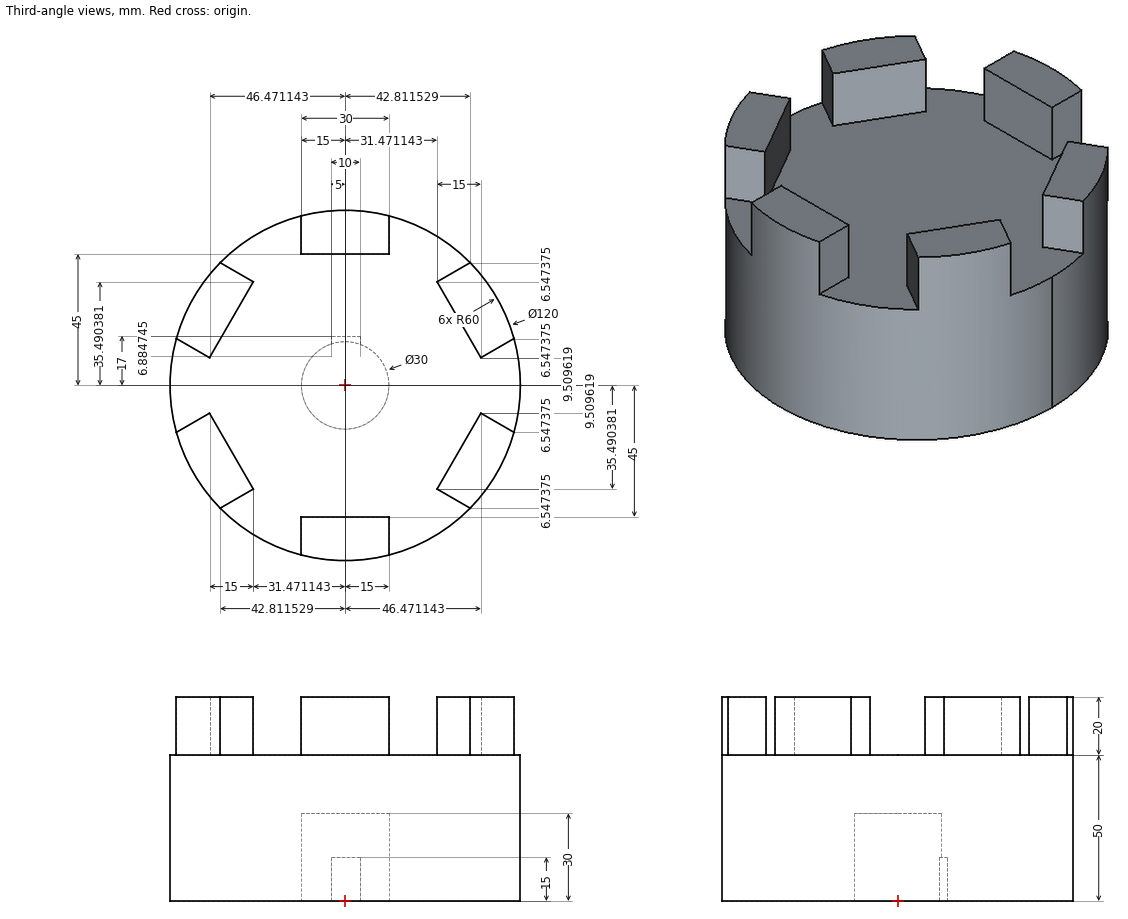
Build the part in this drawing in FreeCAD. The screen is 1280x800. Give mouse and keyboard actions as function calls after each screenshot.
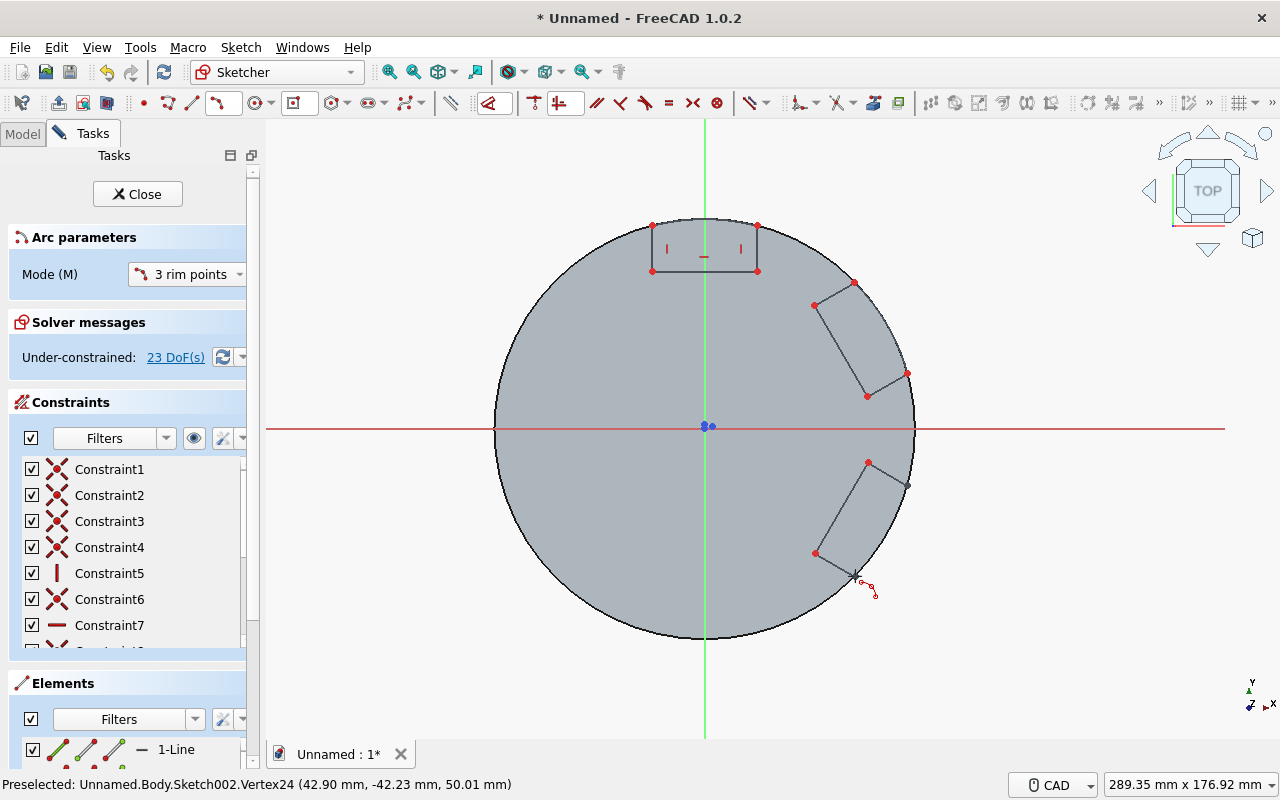
click(855, 577)
click(907, 486)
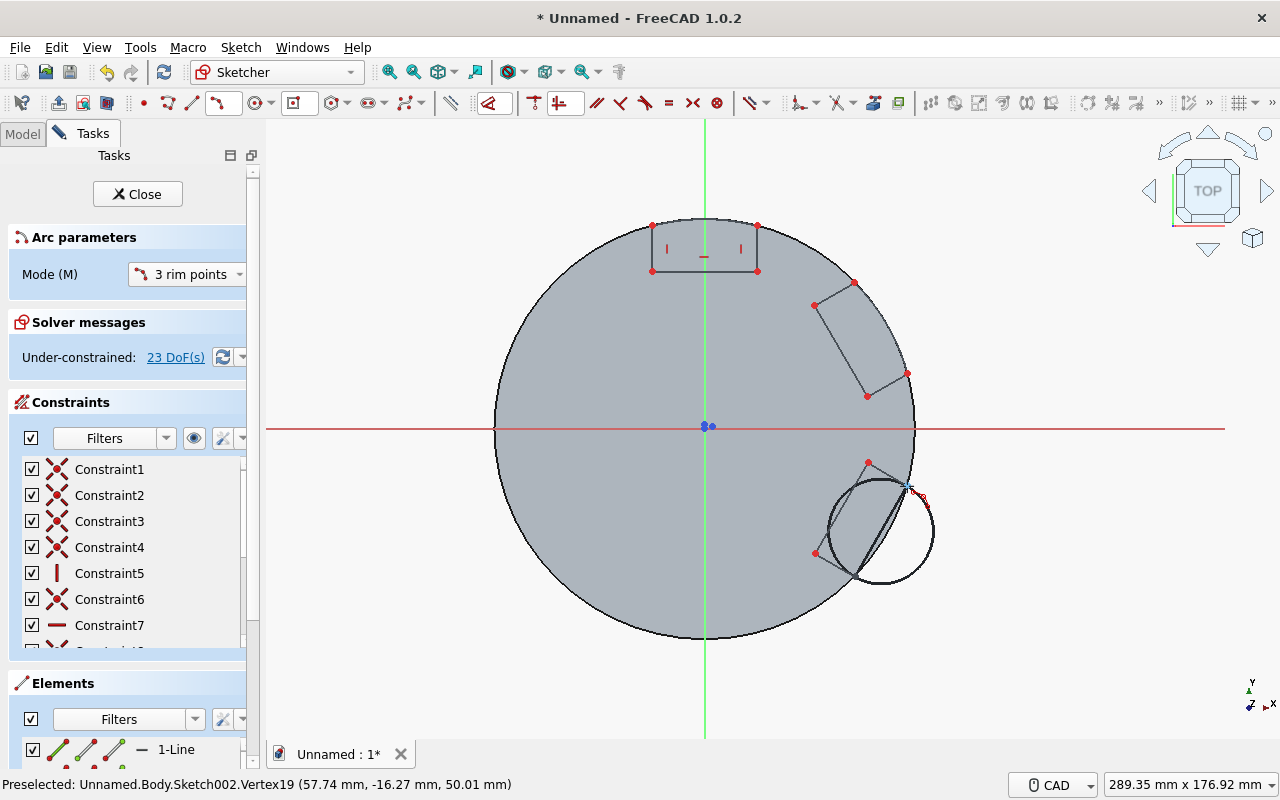
scroll(887, 534, up, 5)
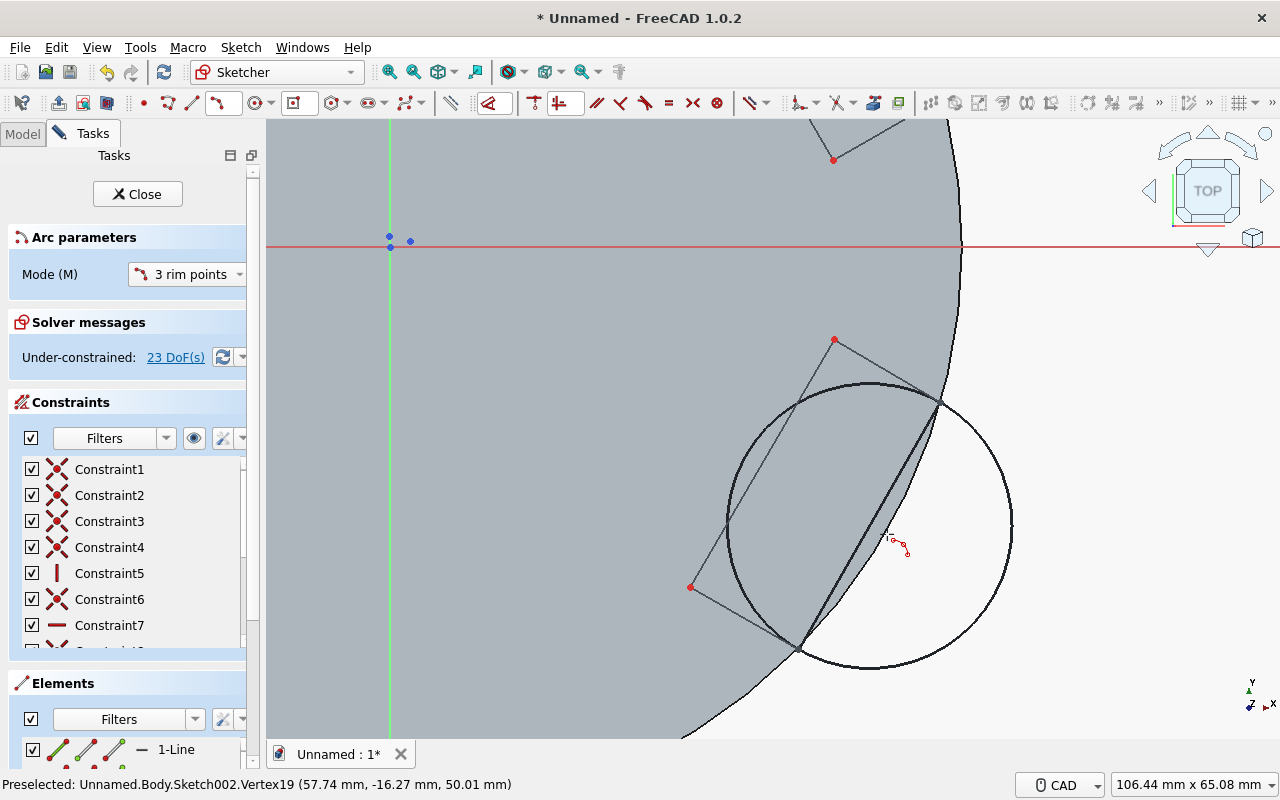
click(885, 533)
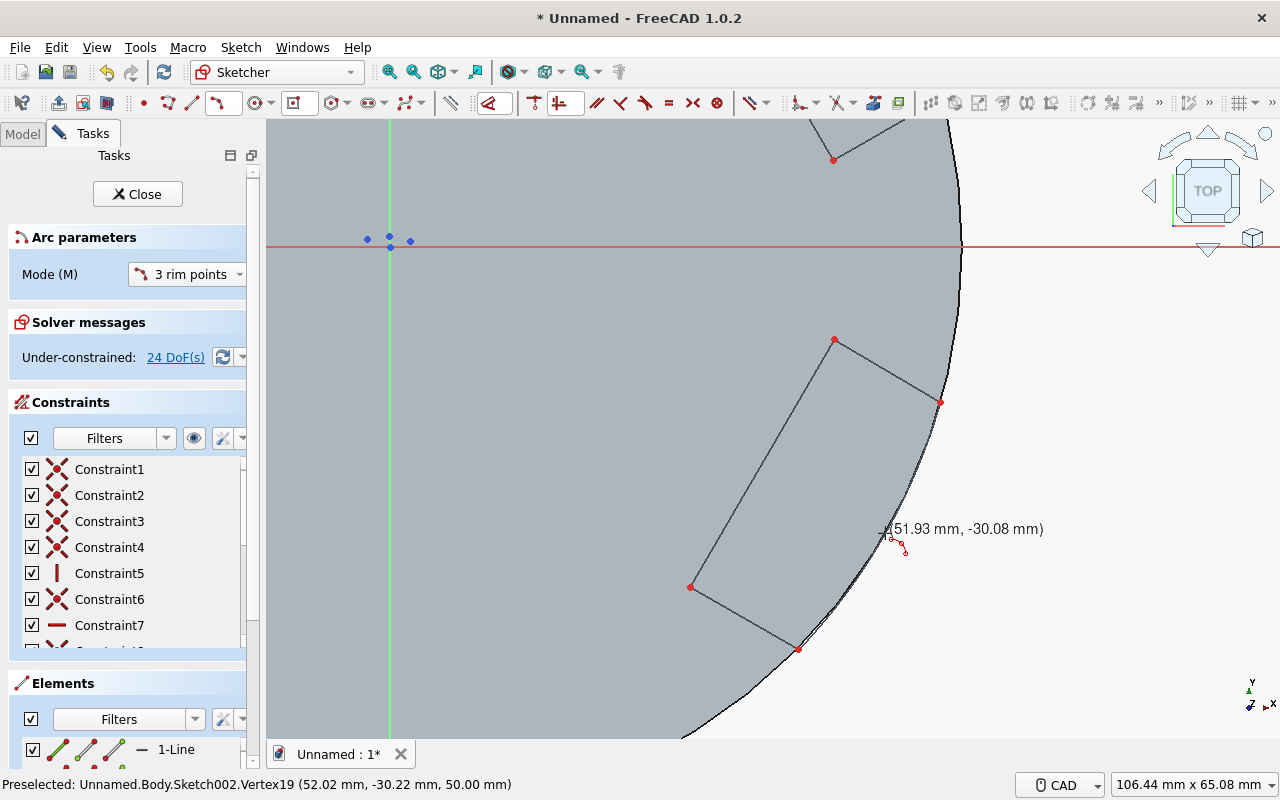
key(g)
key(m)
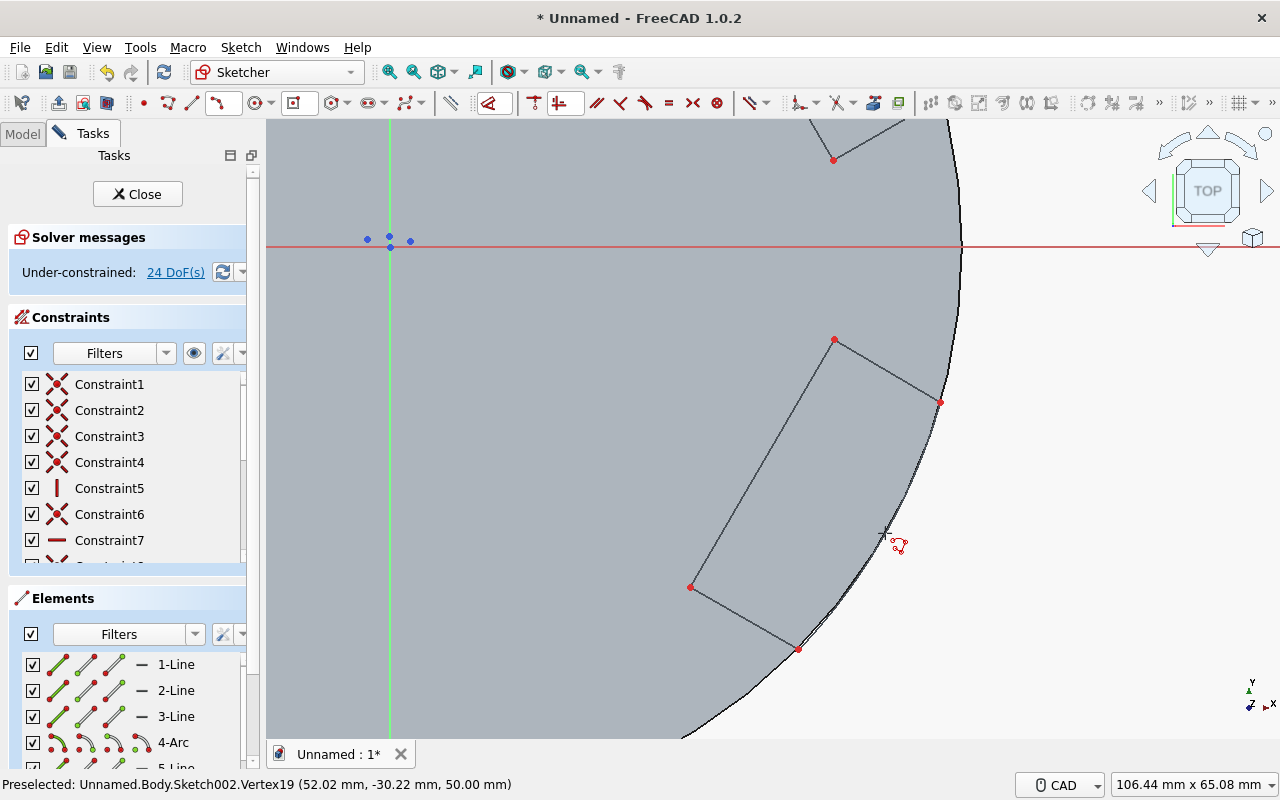
scroll(887, 535, down, 5)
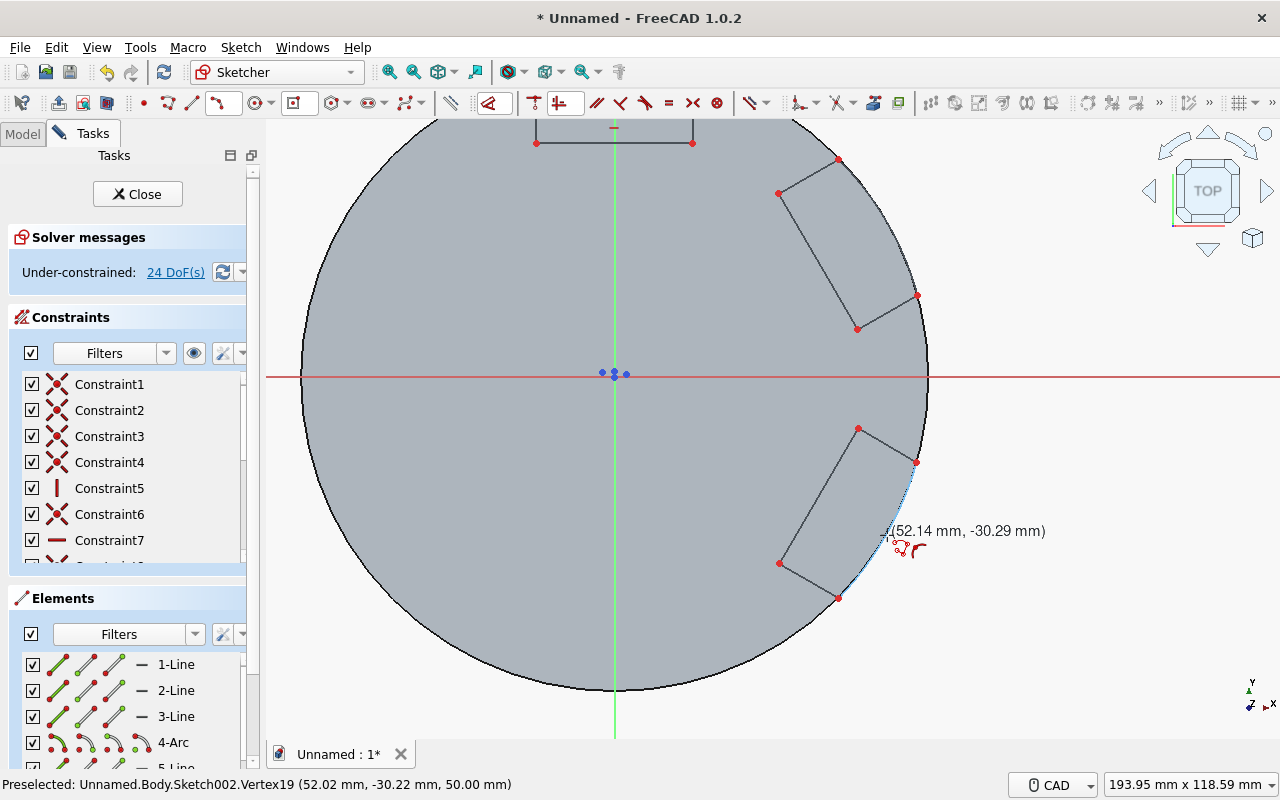
click(757, 633)
click(757, 587)
click(652, 587)
click(652, 633)
right_click(652, 633)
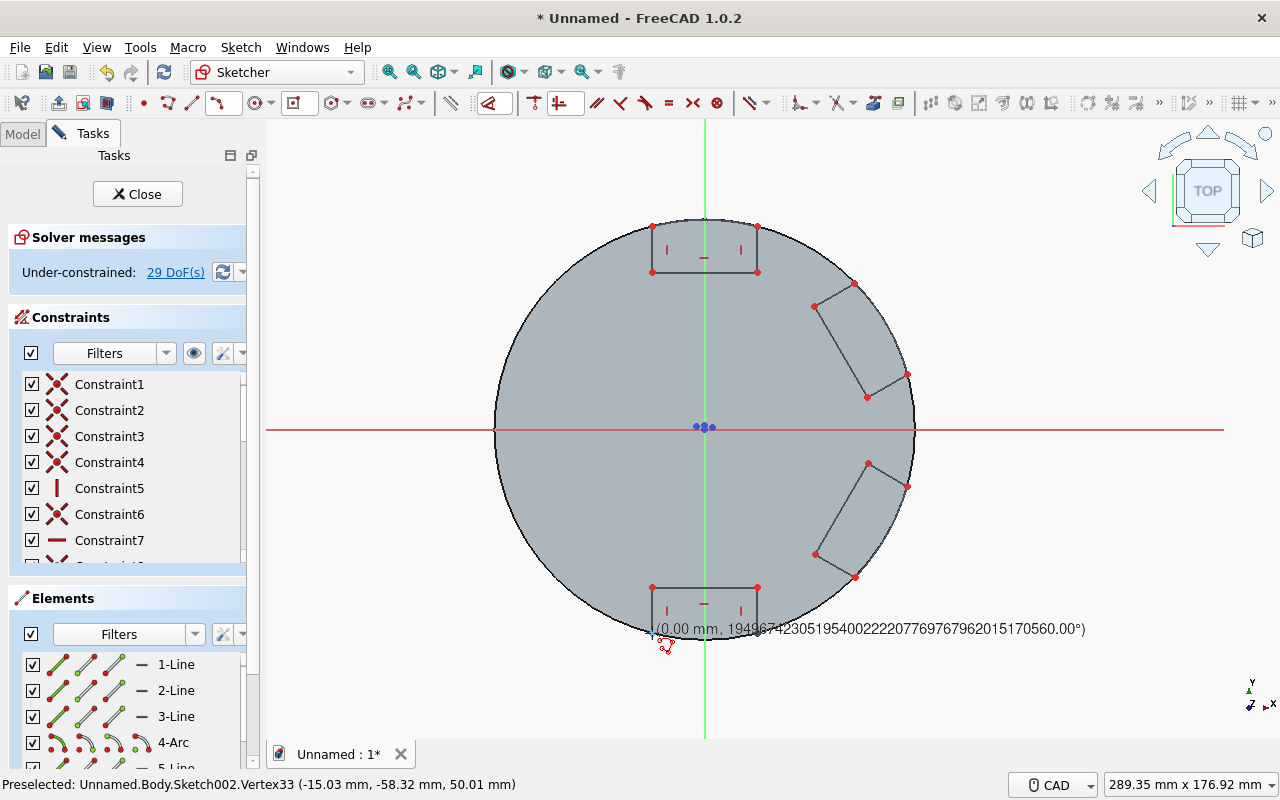
click(218, 104)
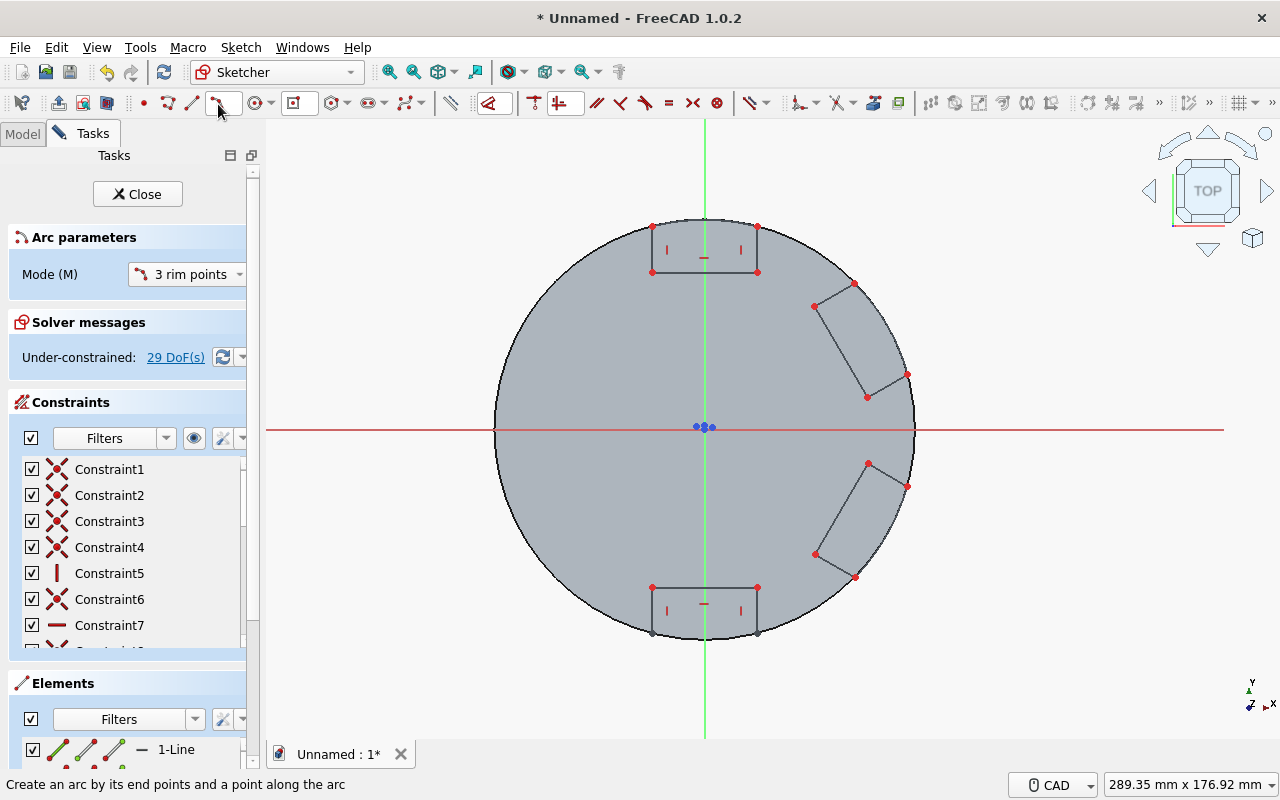
click(652, 634)
click(757, 634)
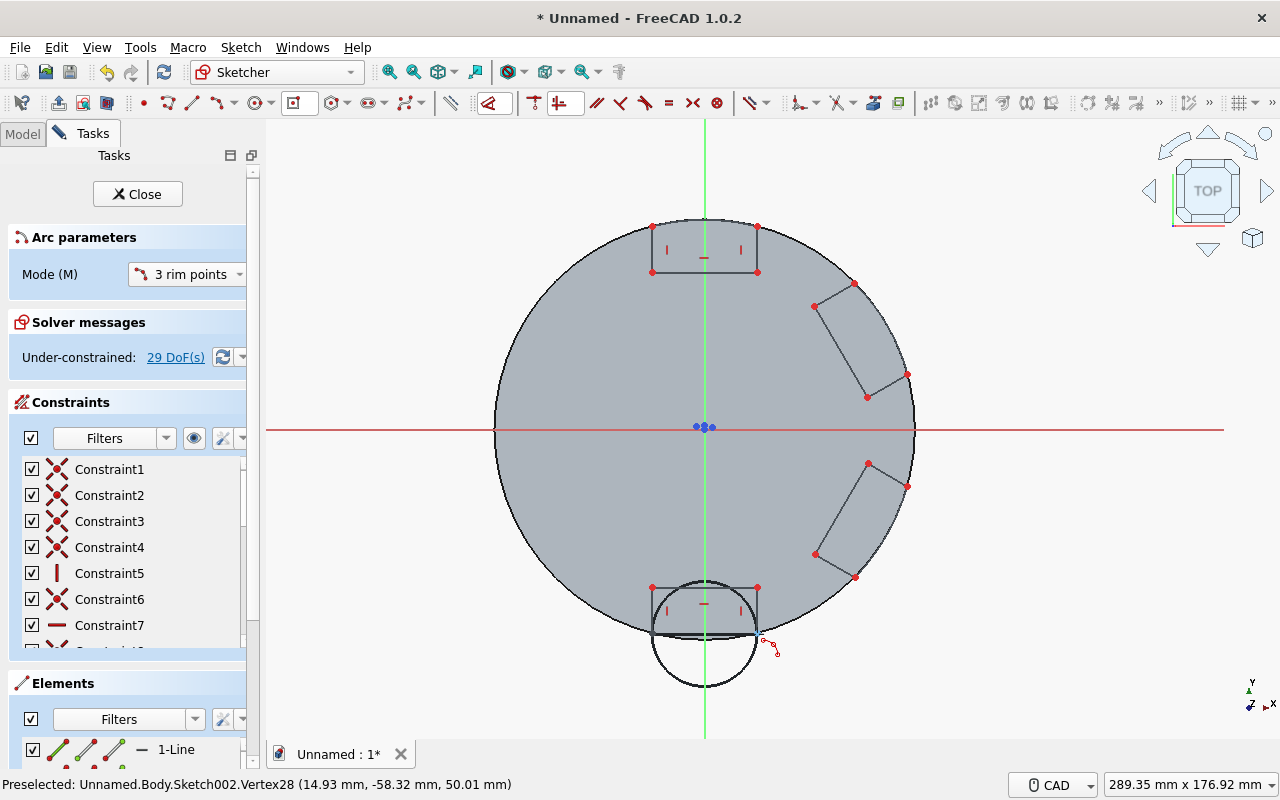
scroll(694, 640, up, 5)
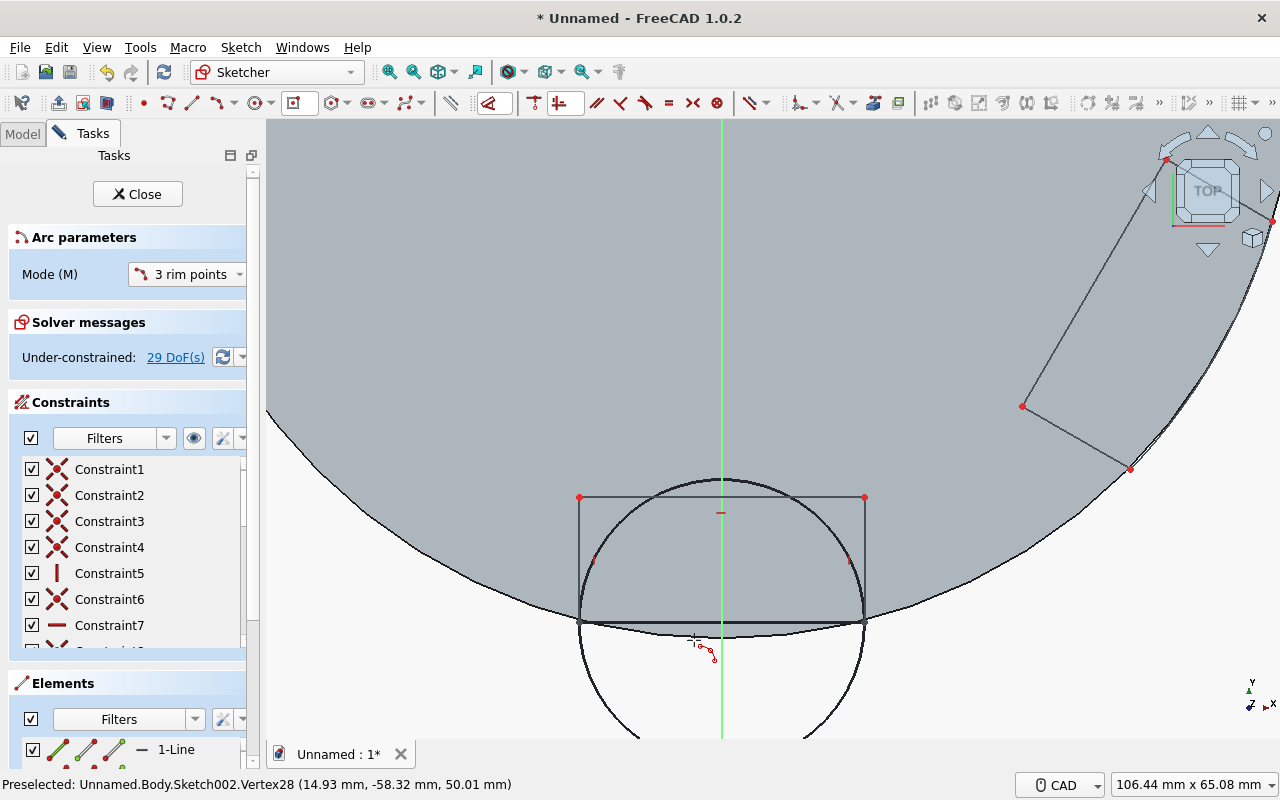
click(693, 638)